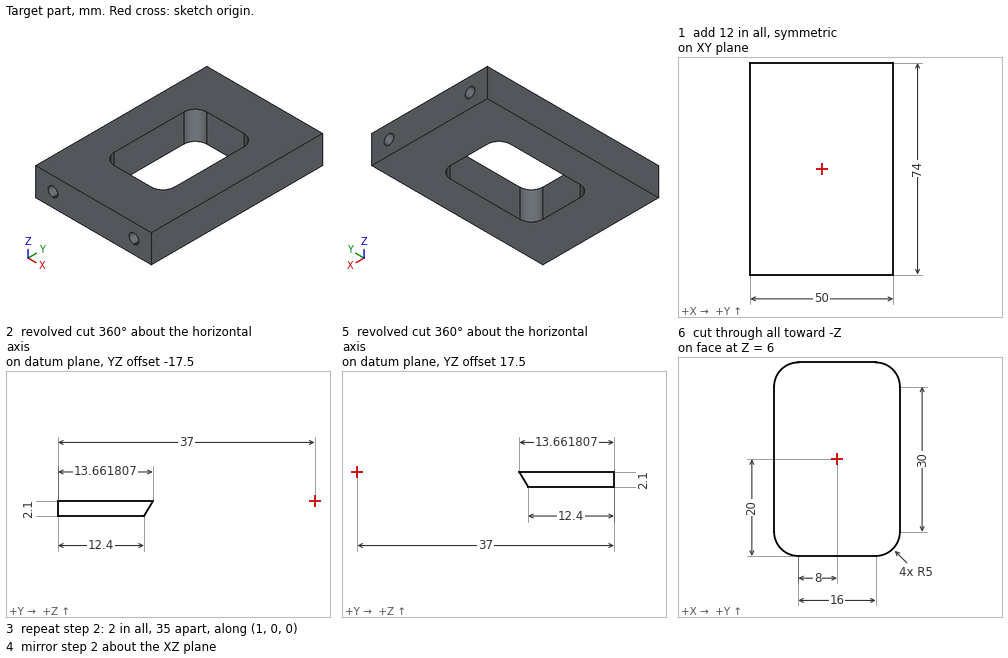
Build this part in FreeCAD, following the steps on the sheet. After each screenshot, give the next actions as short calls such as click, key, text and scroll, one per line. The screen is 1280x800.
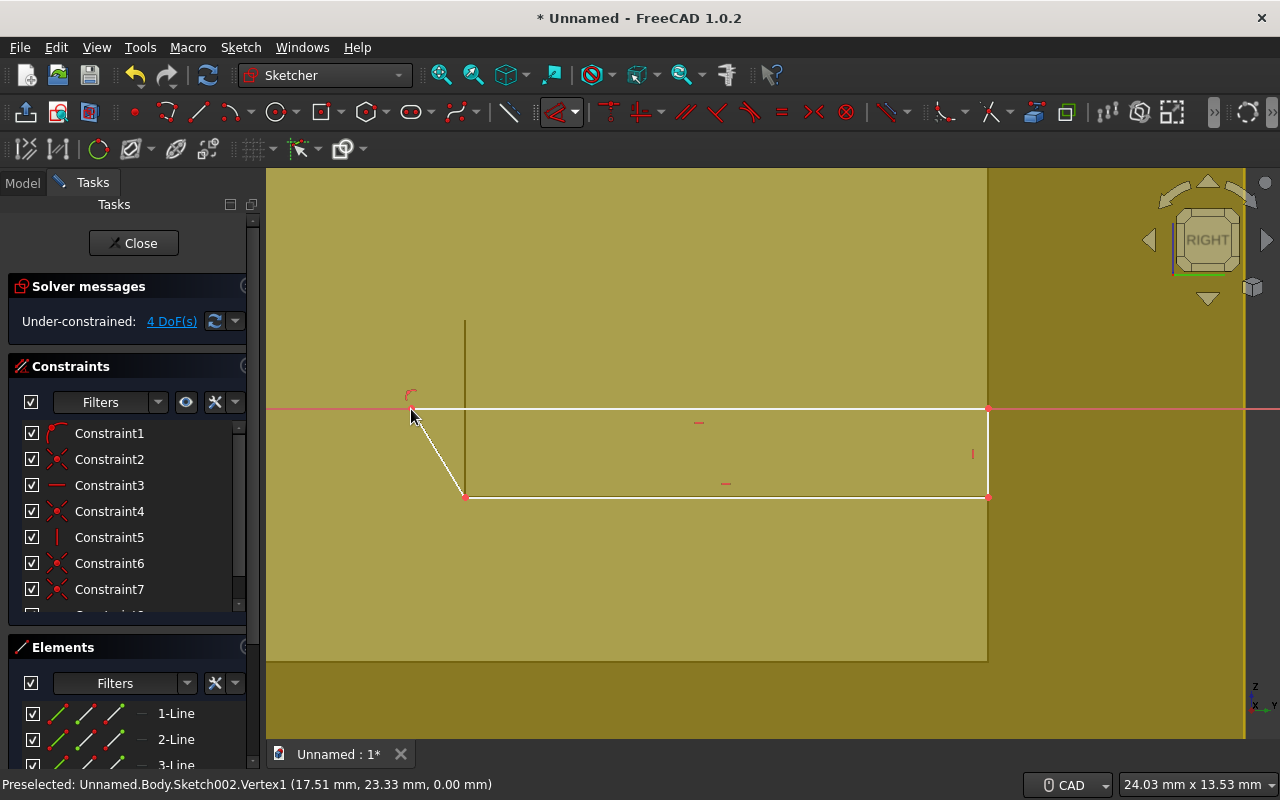
click(988, 471)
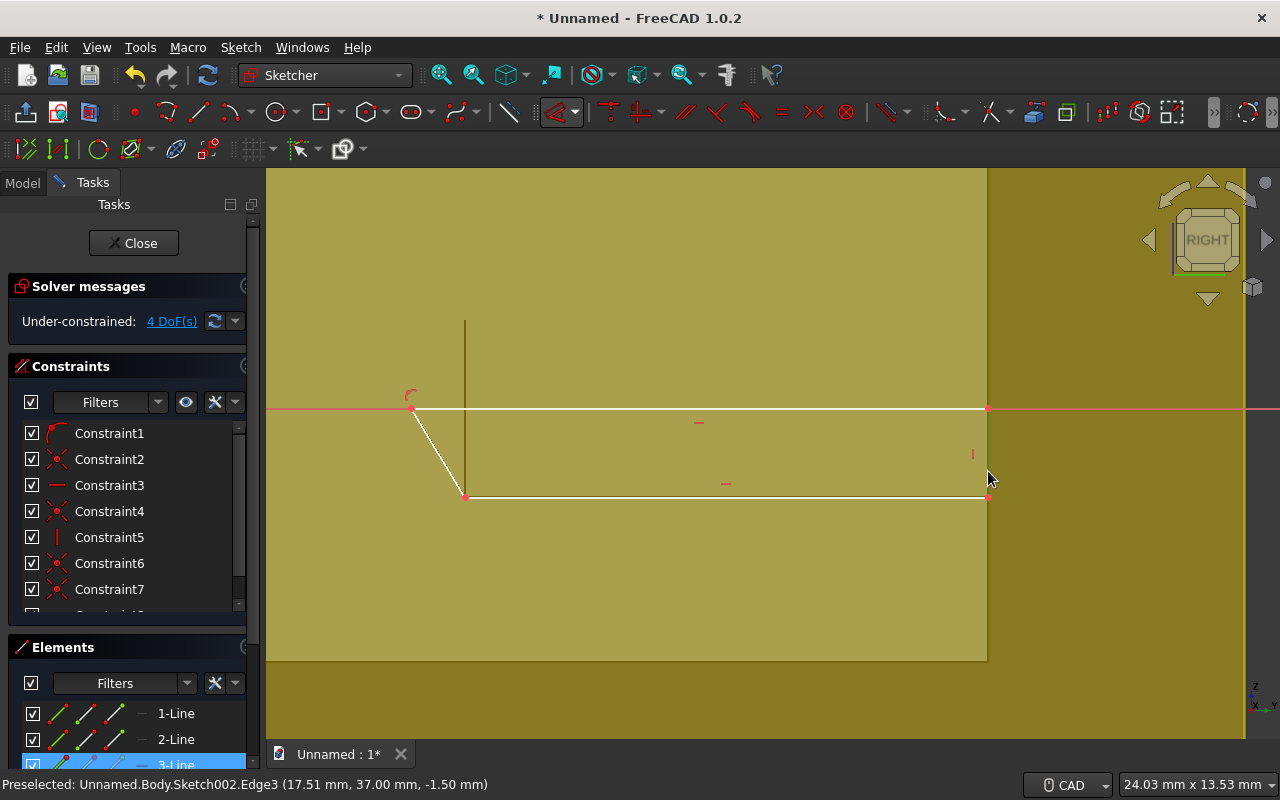
key(i)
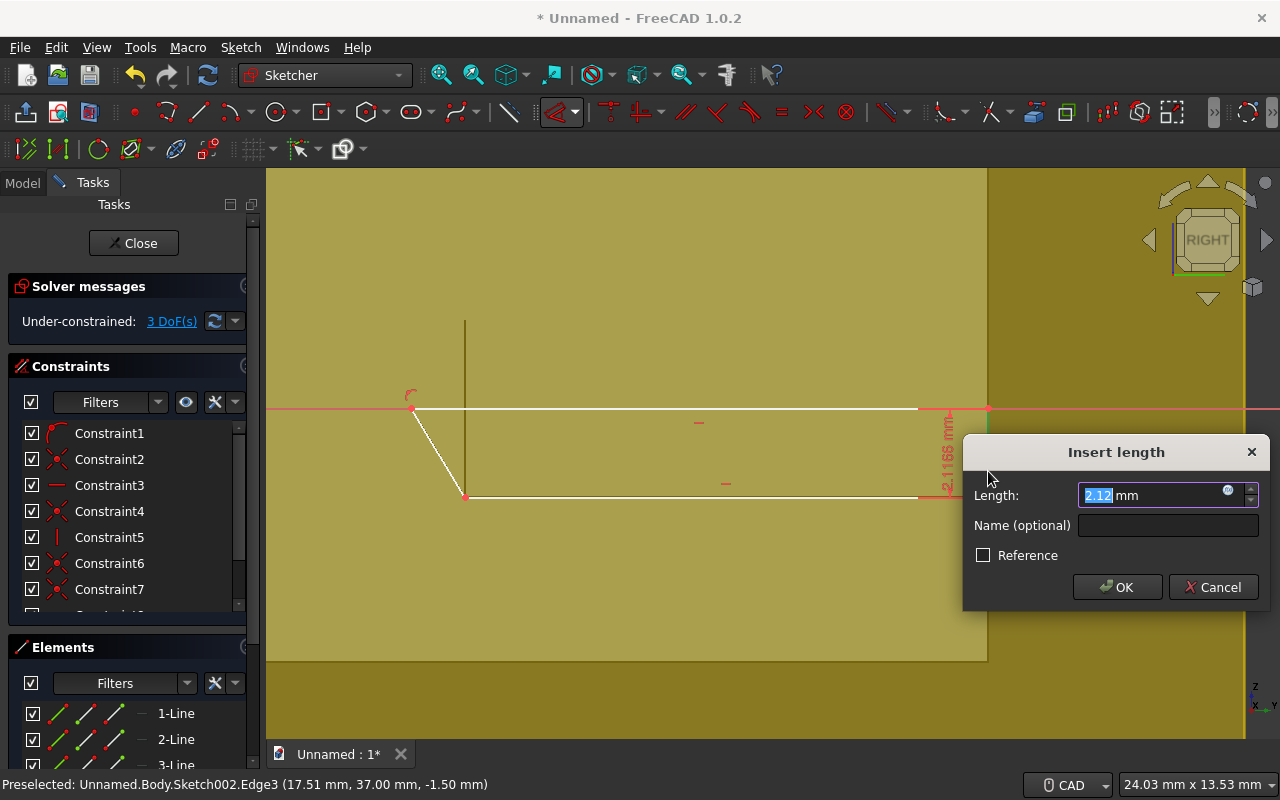
text(2.1)
key(Return)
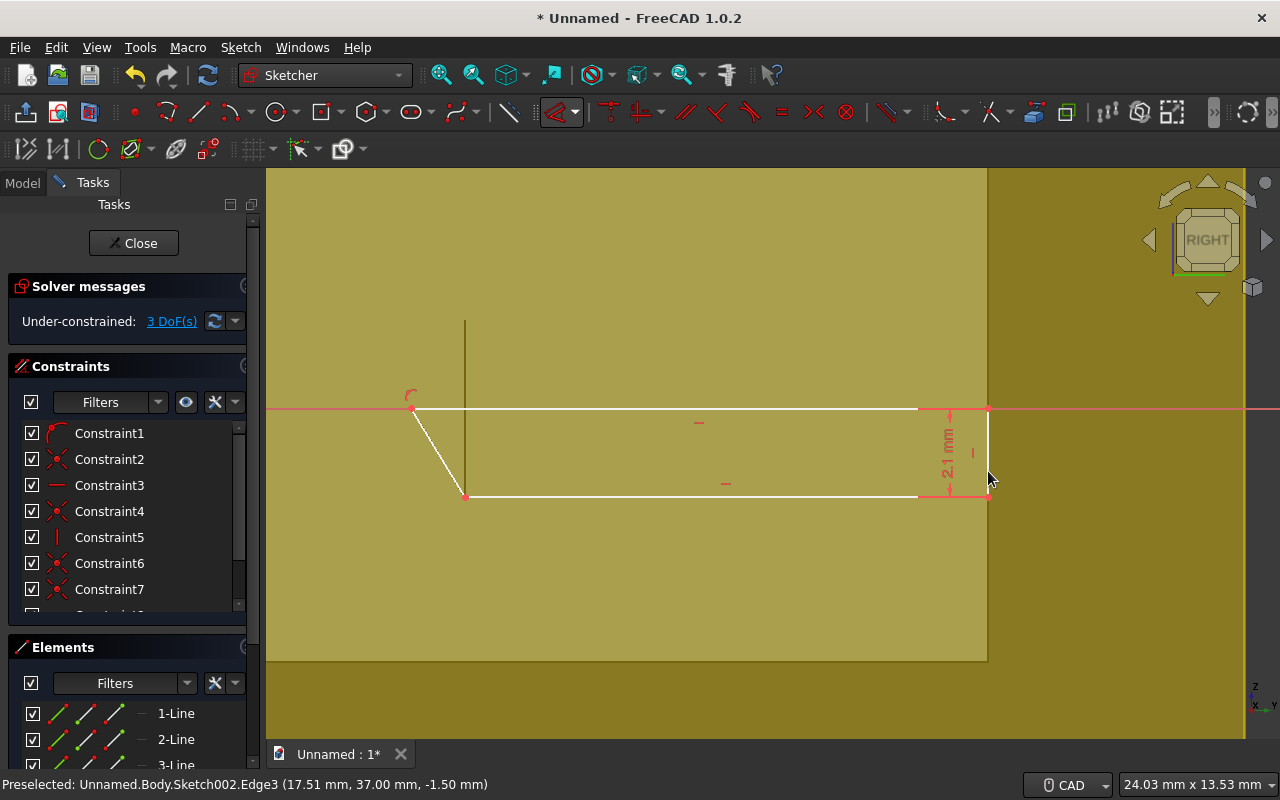
click(988, 497)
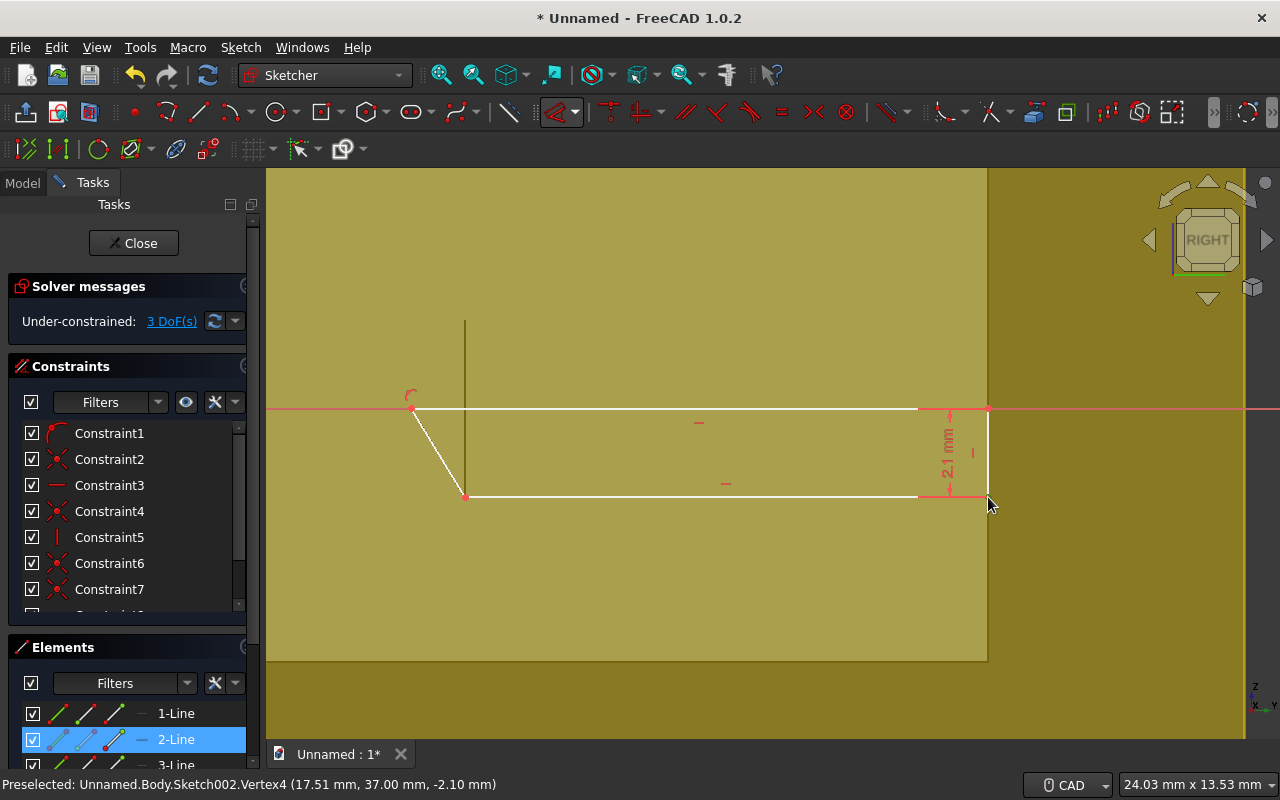
key(l)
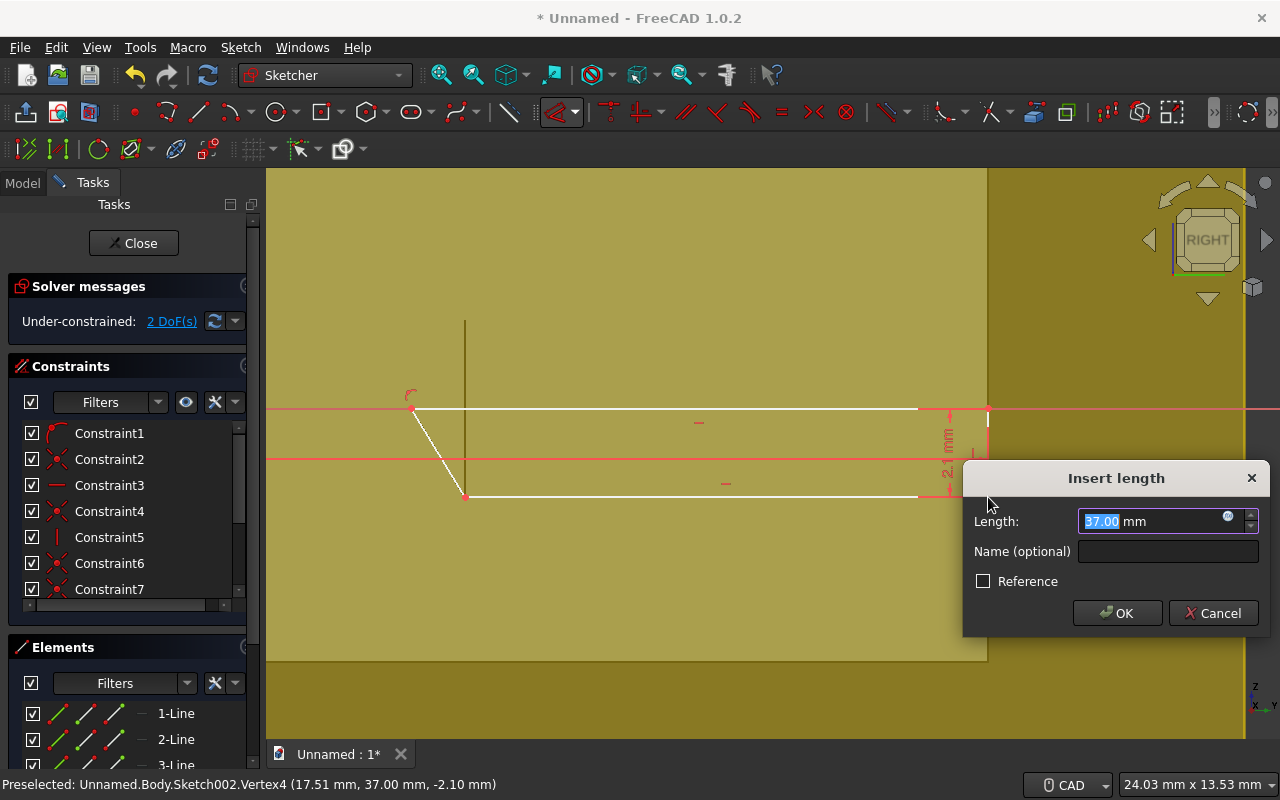
text(37)
key(Return)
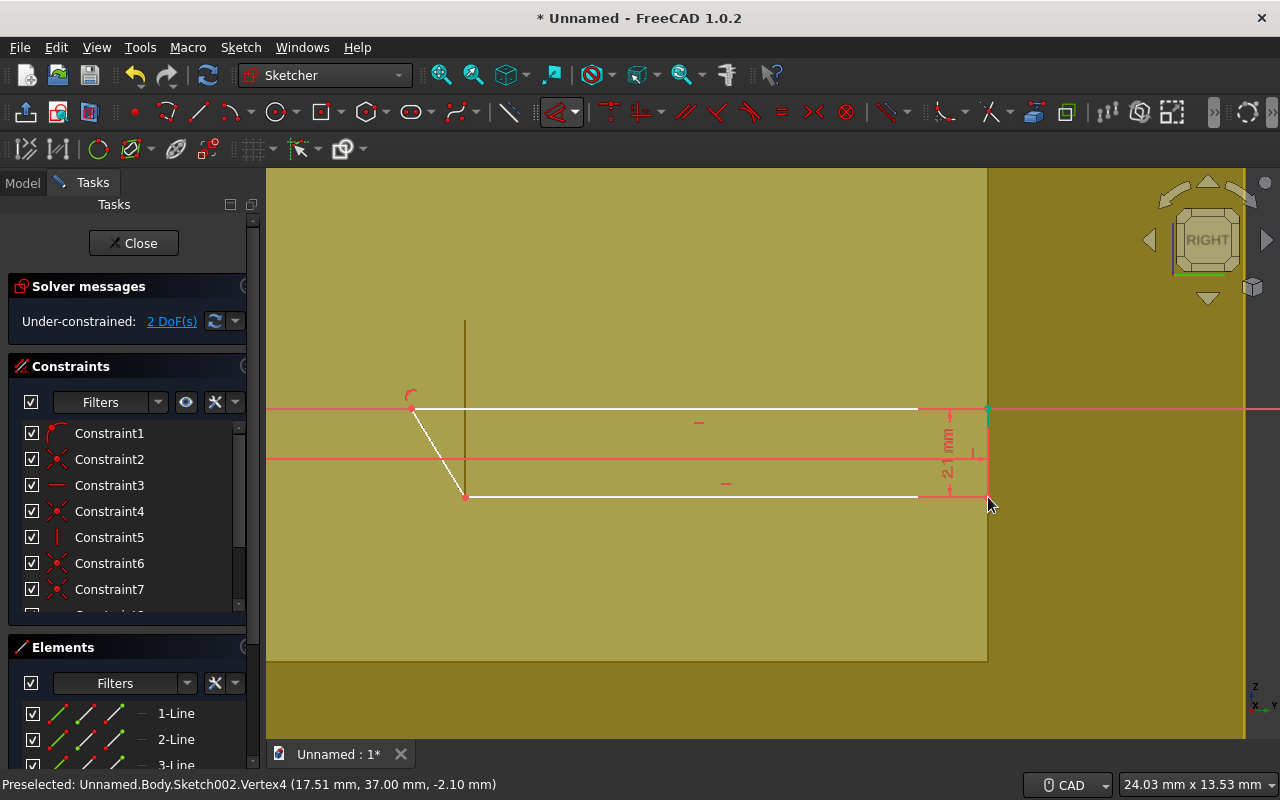
click(622, 497)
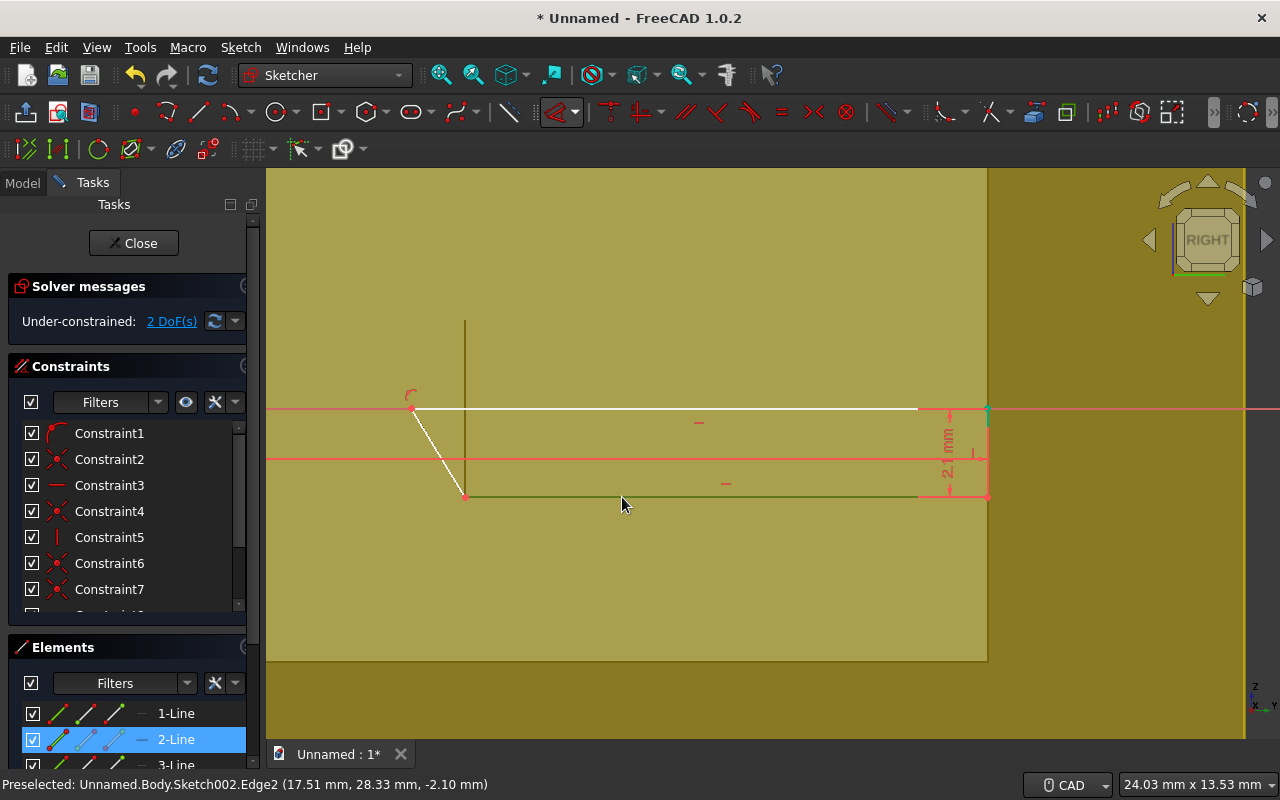
click(578, 112)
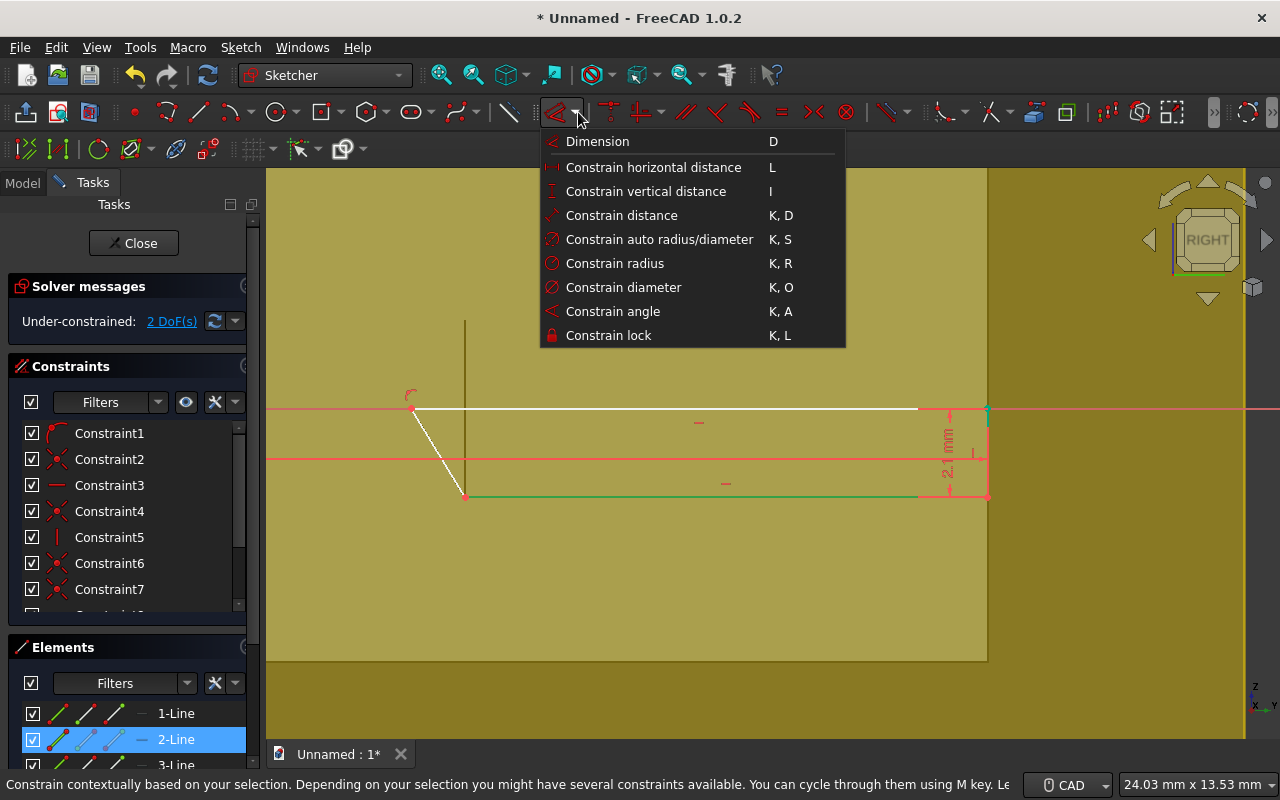
click(693, 167)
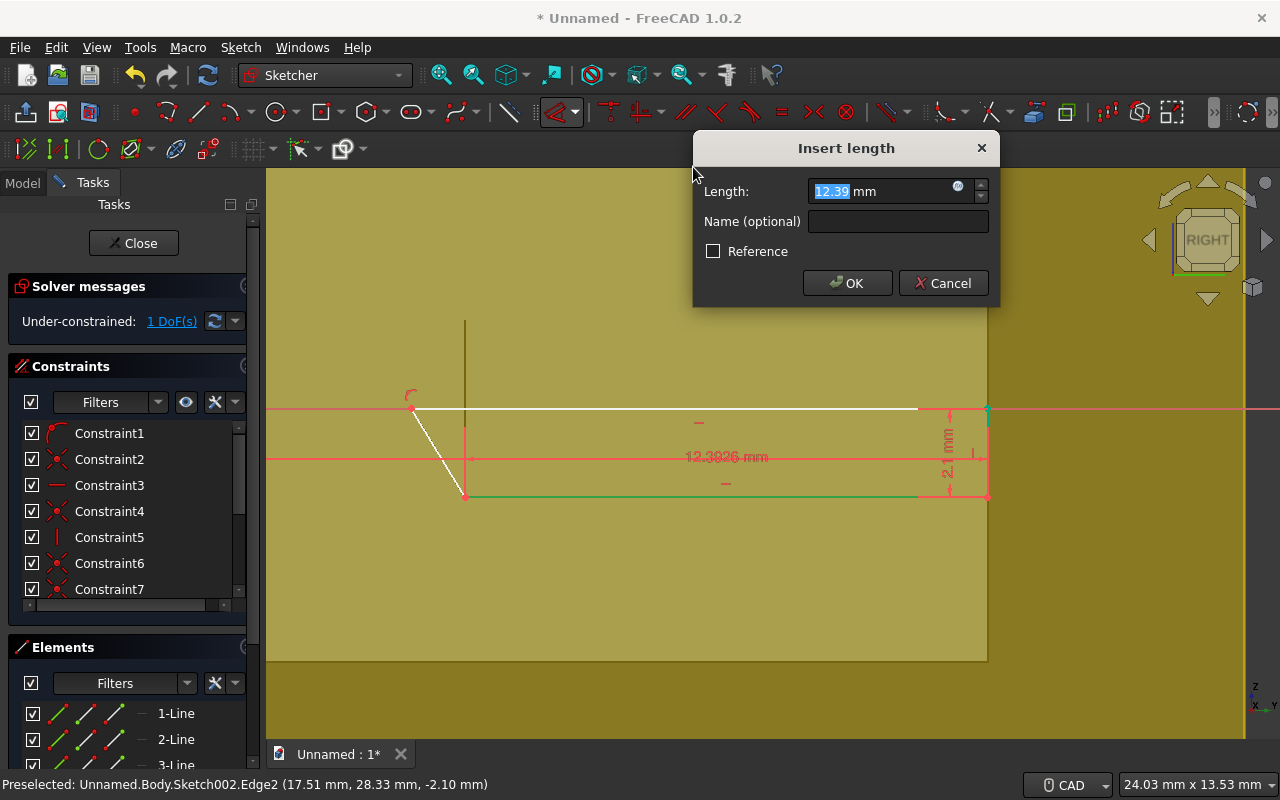
text(12.4)
key(Return)